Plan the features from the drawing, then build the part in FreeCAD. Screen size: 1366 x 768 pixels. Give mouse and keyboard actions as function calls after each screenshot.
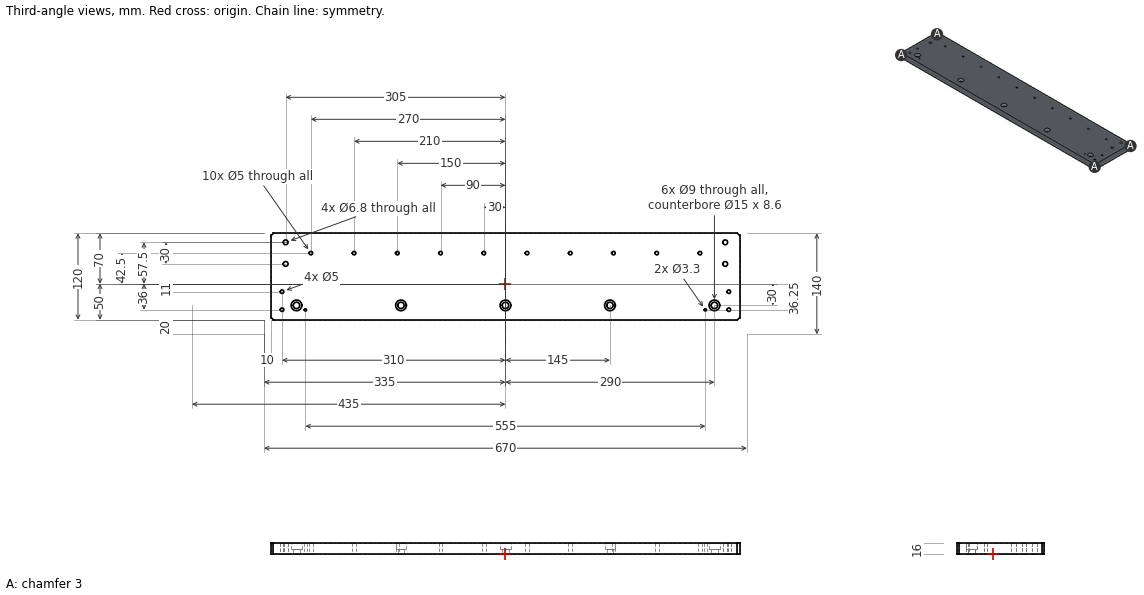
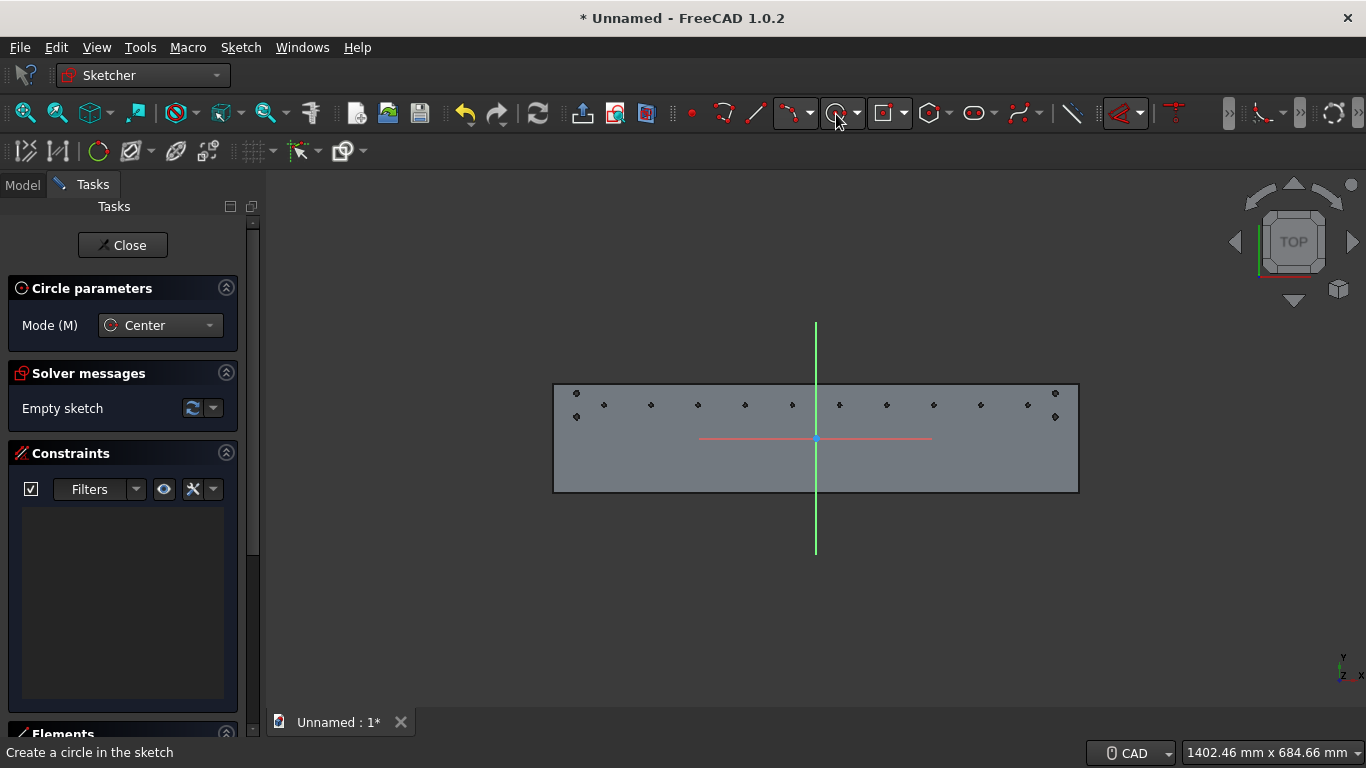
scroll(1043, 462, up, 10)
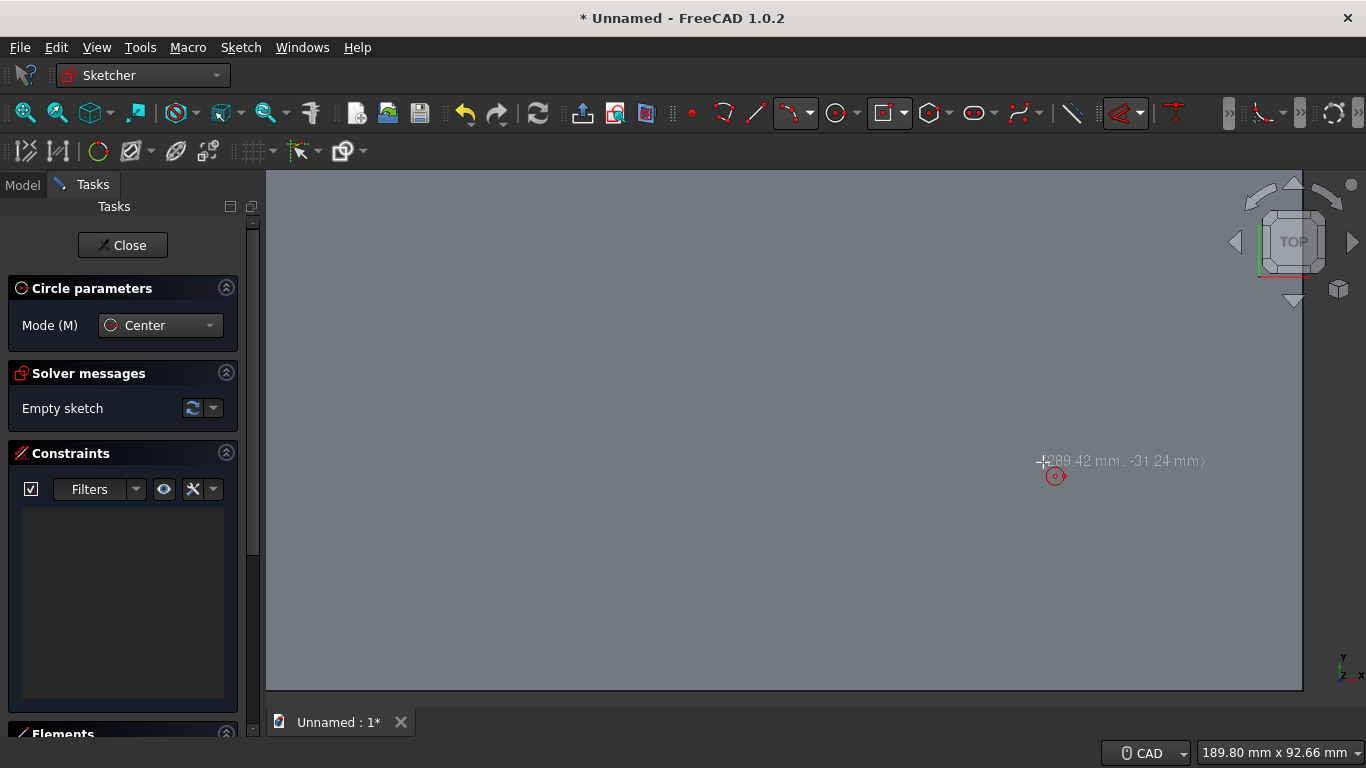
scroll(1105, 449, down, 9)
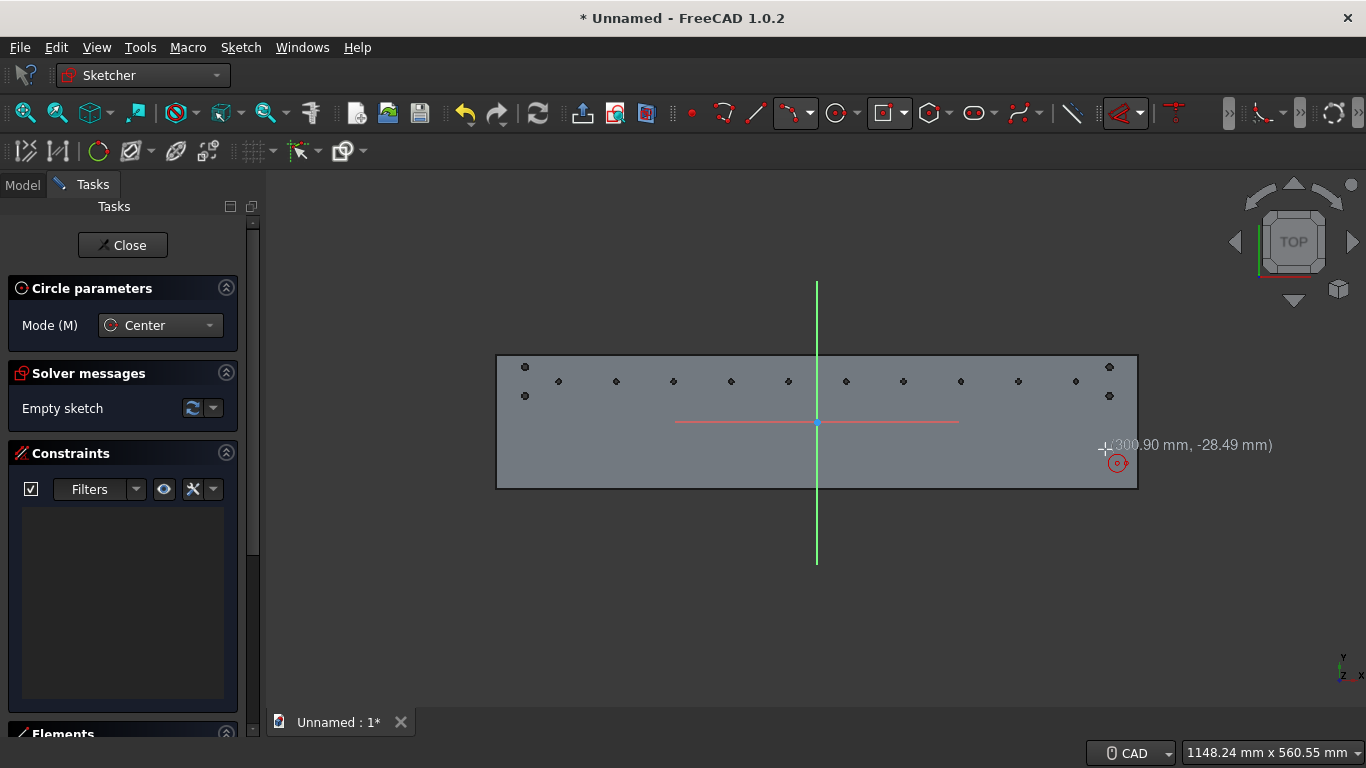
click(1095, 451)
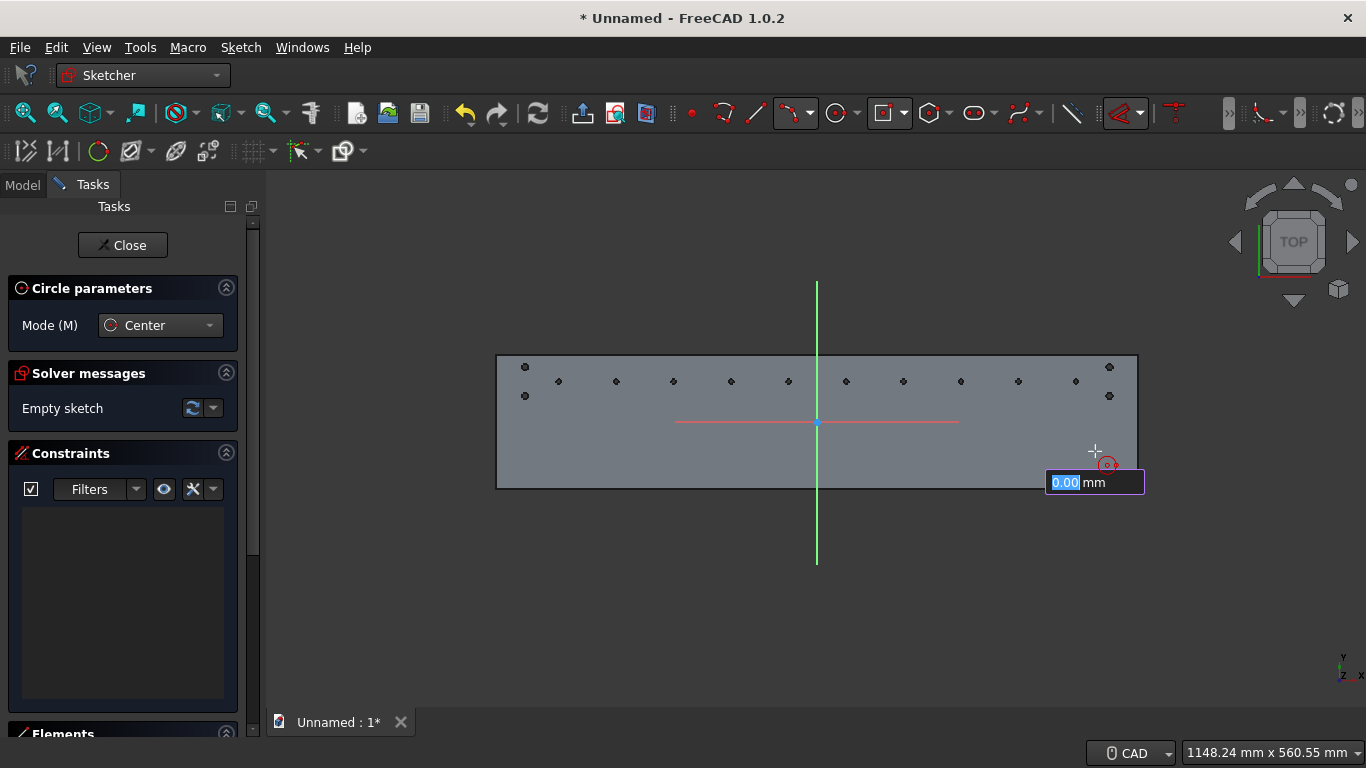
scroll(1098, 448, up, 7)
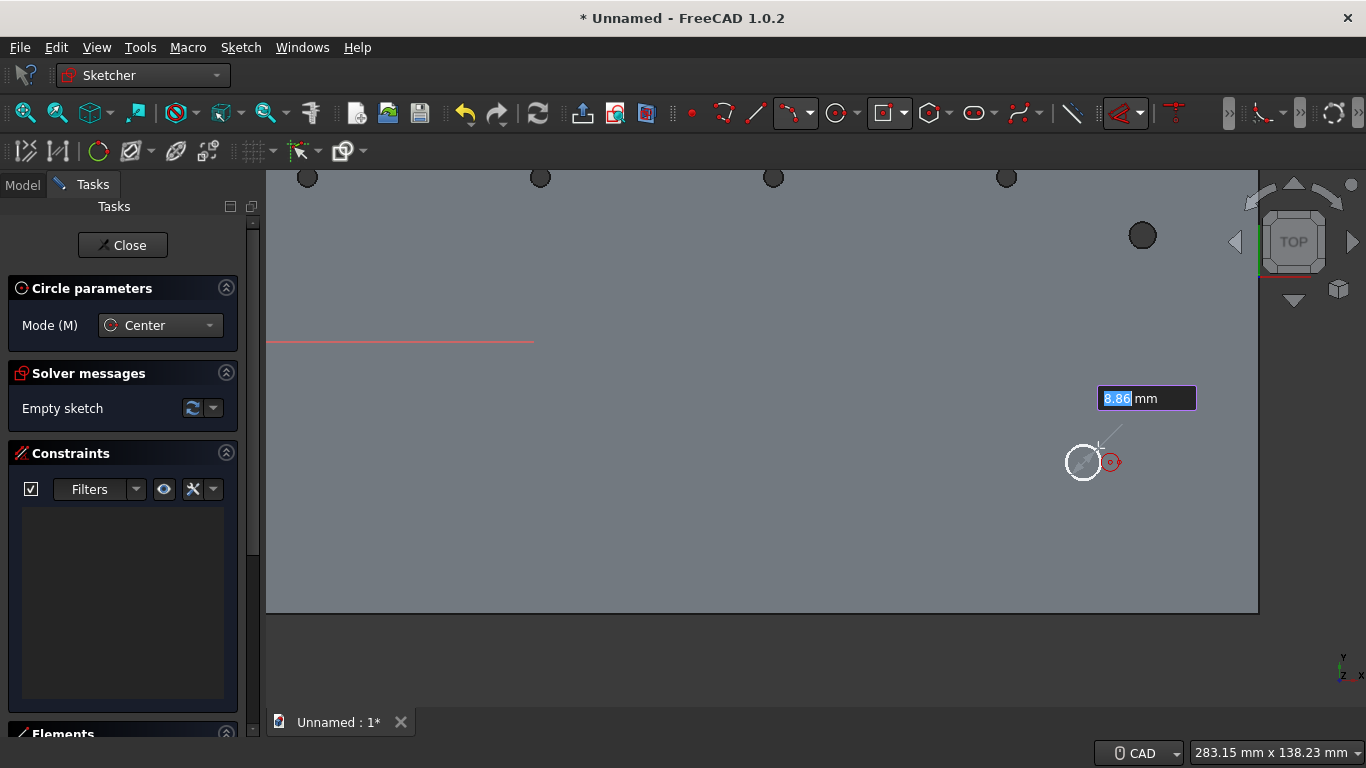
click(1097, 446)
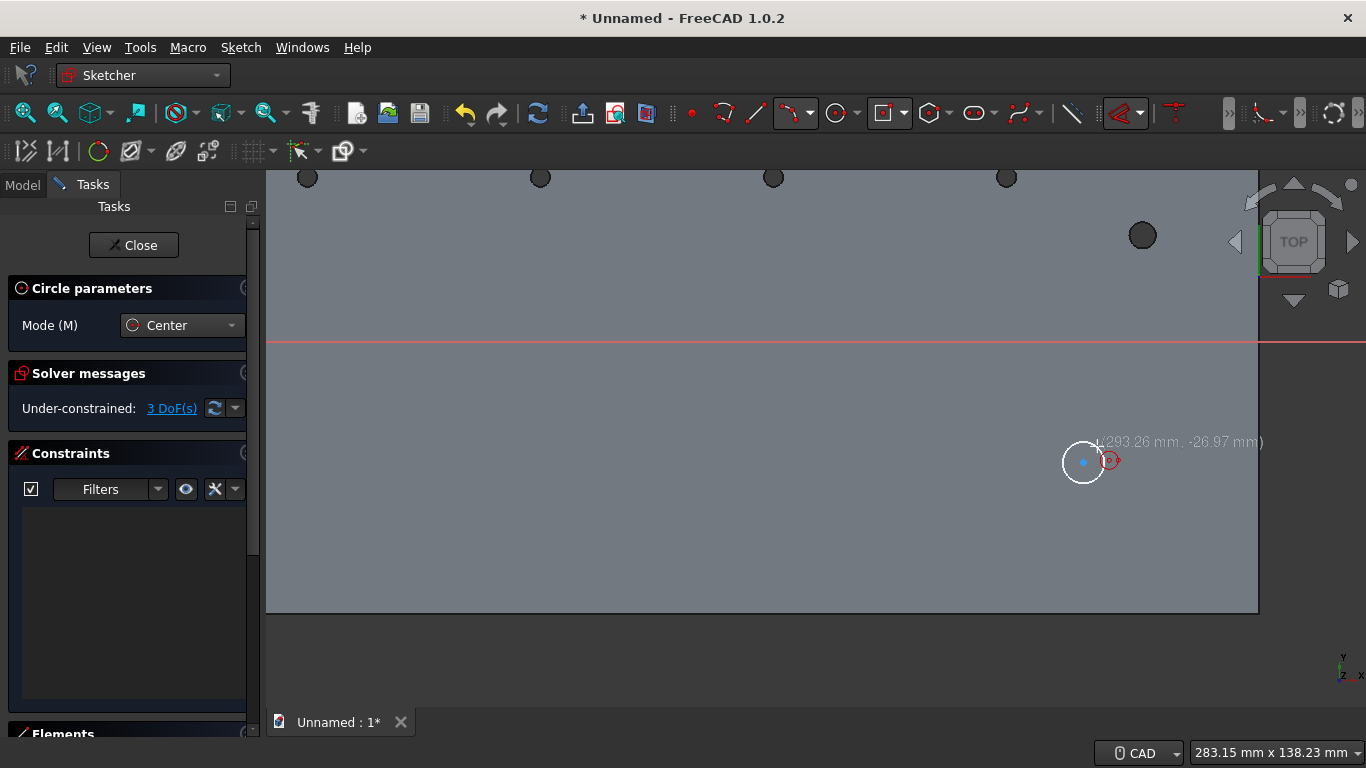
scroll(521, 459, up, 2)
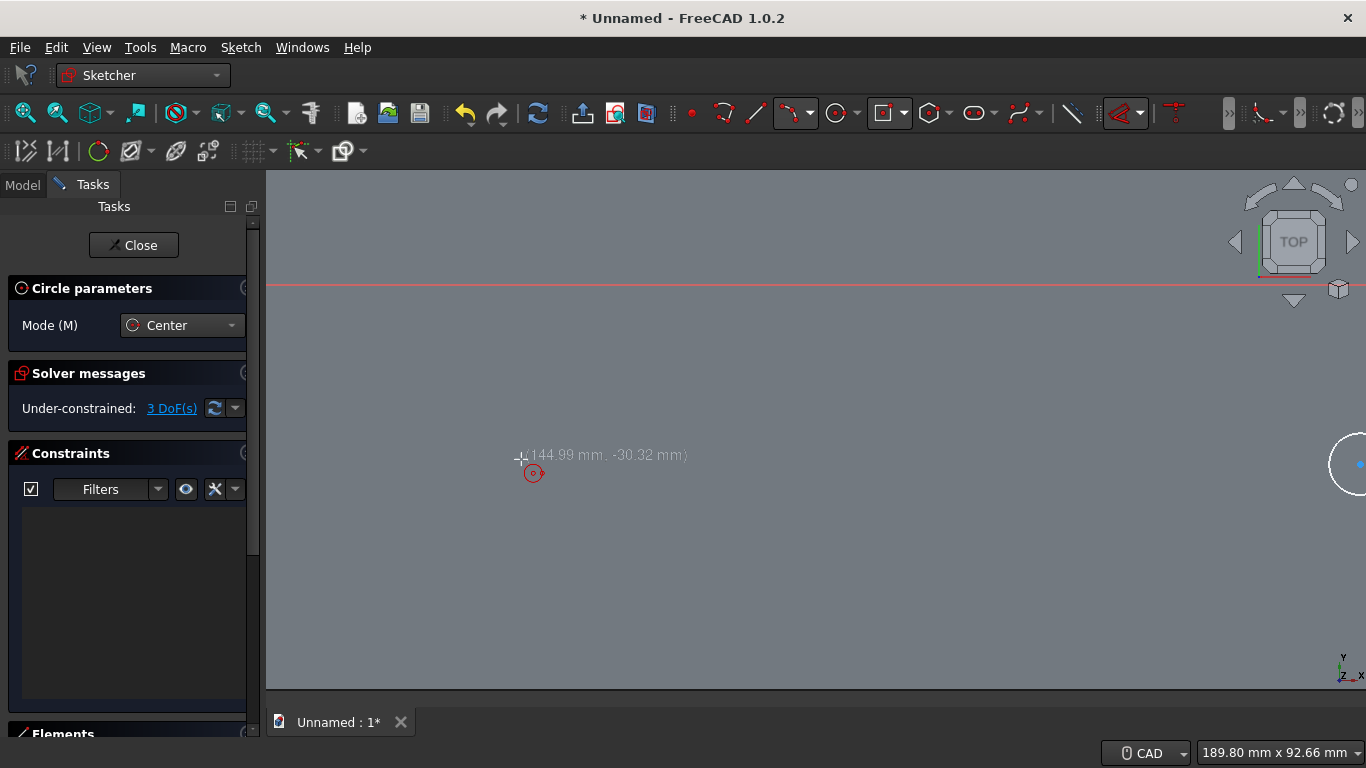
scroll(1042, 449, down, 9)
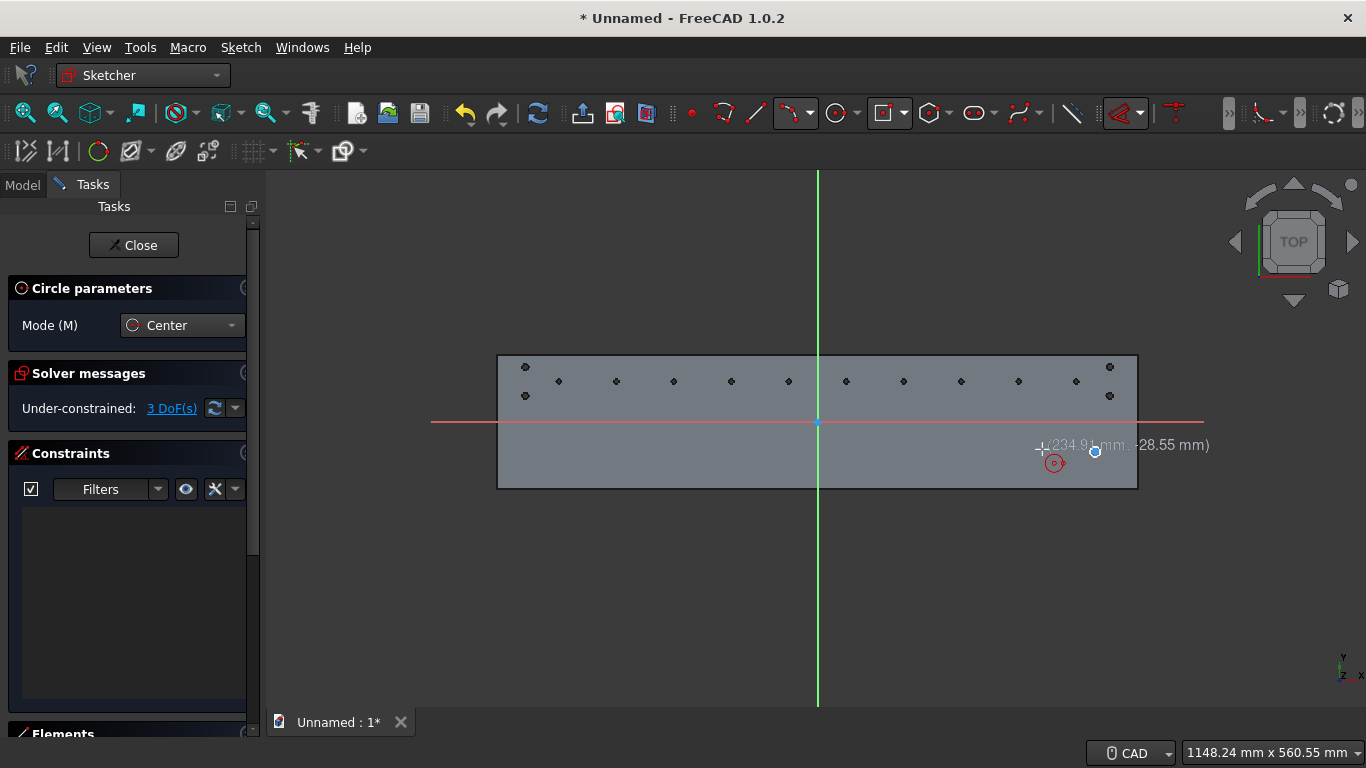
click(956, 451)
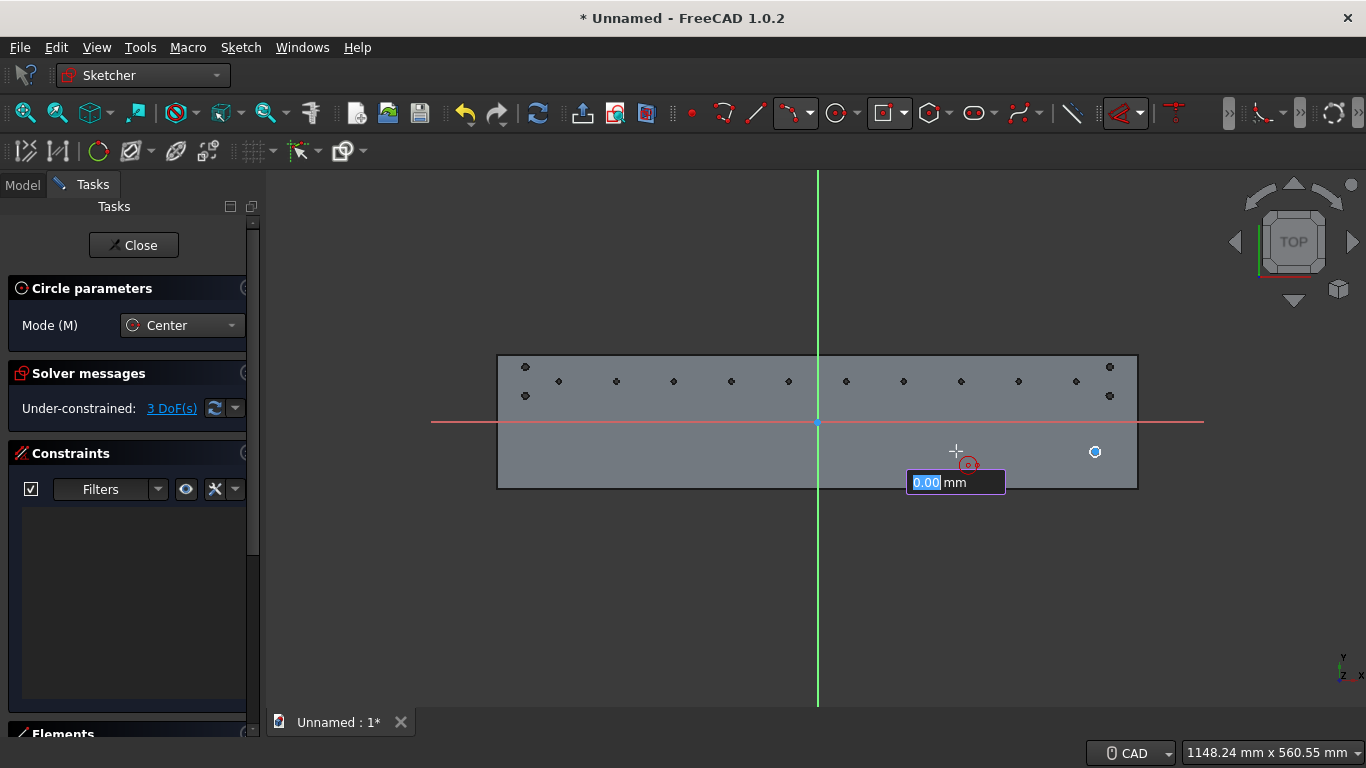
scroll(960, 448, up, 7)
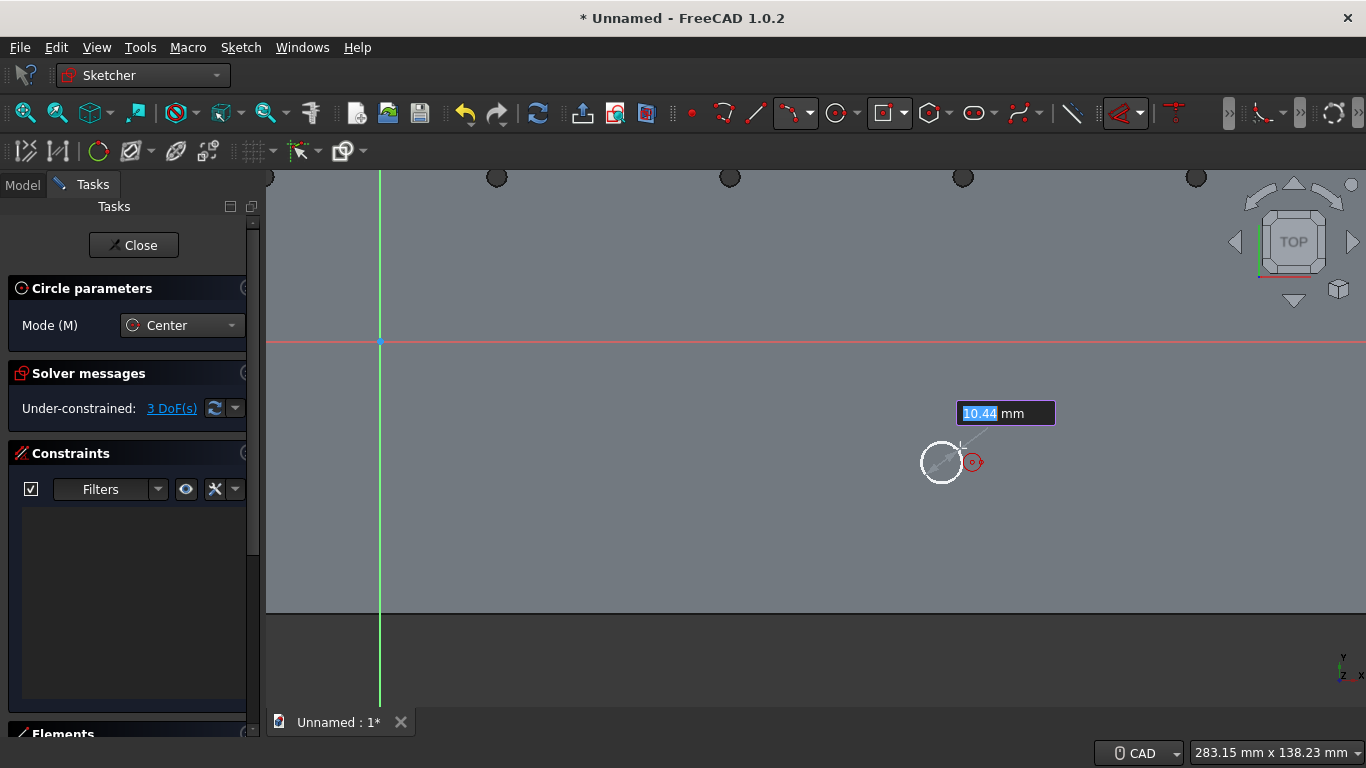
click(956, 446)